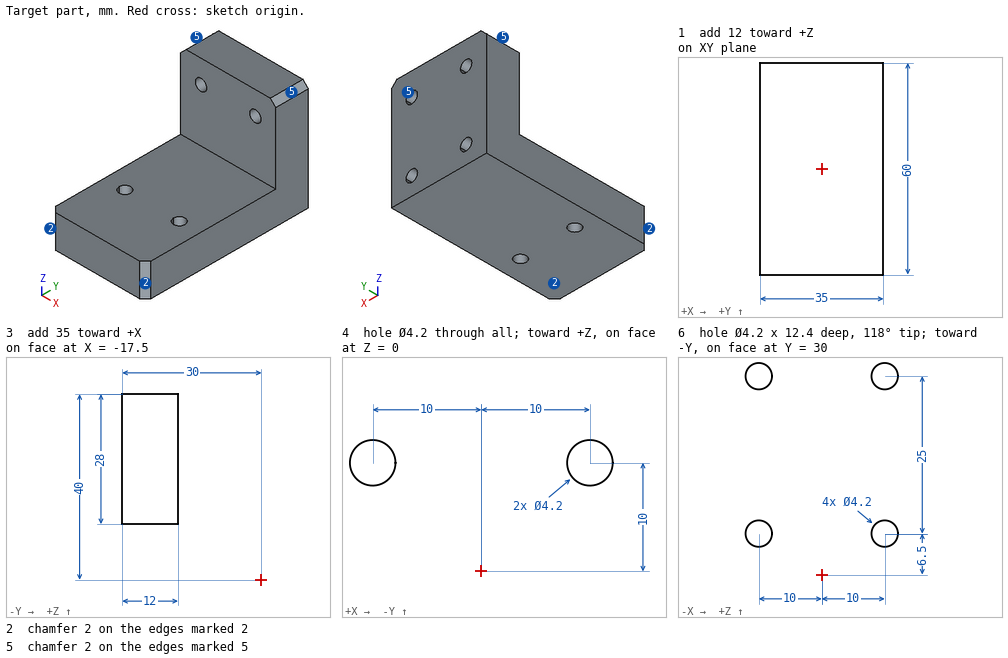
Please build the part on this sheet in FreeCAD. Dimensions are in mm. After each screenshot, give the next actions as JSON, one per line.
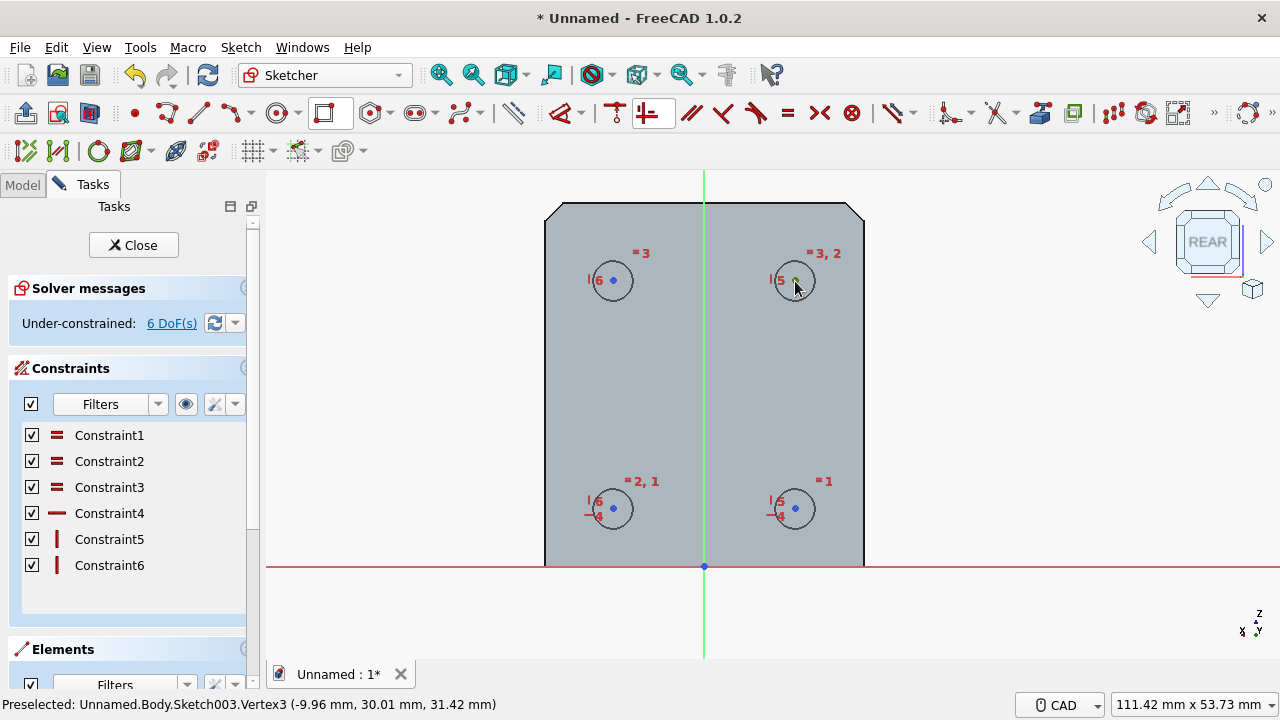
{"action": "left_click", "coordinate": [613, 281]}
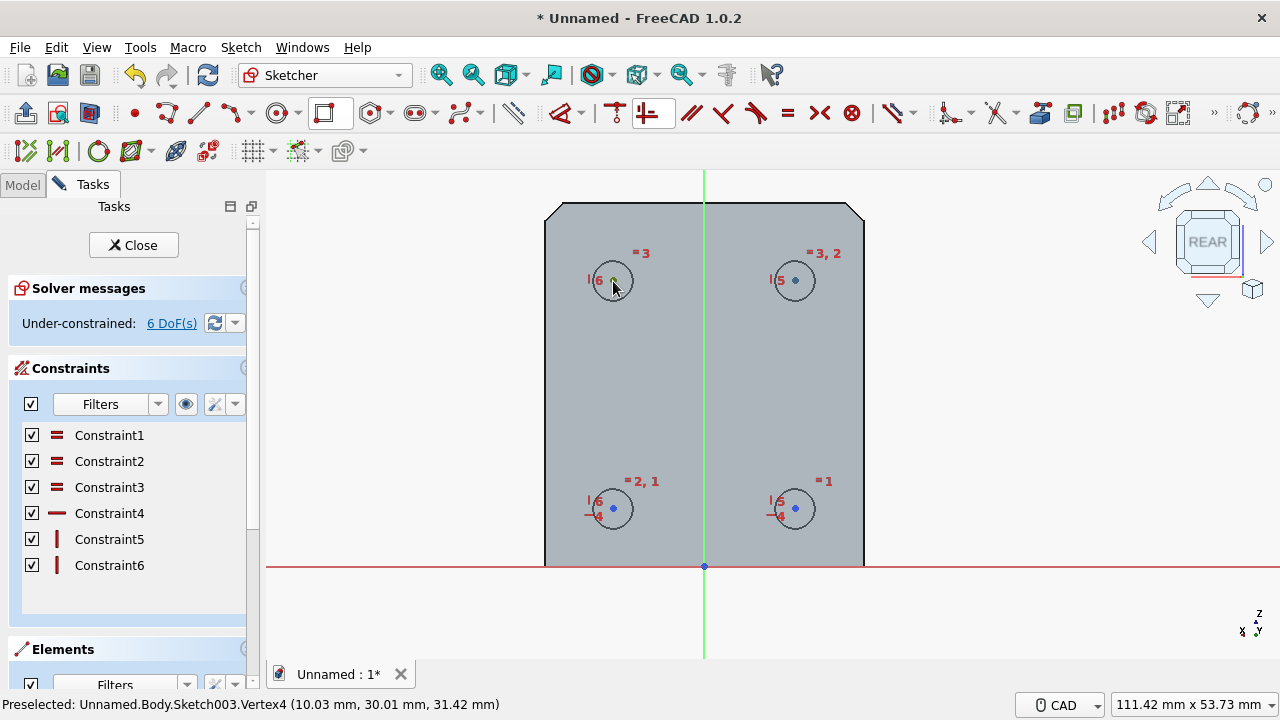
{"action": "key", "text": "h"}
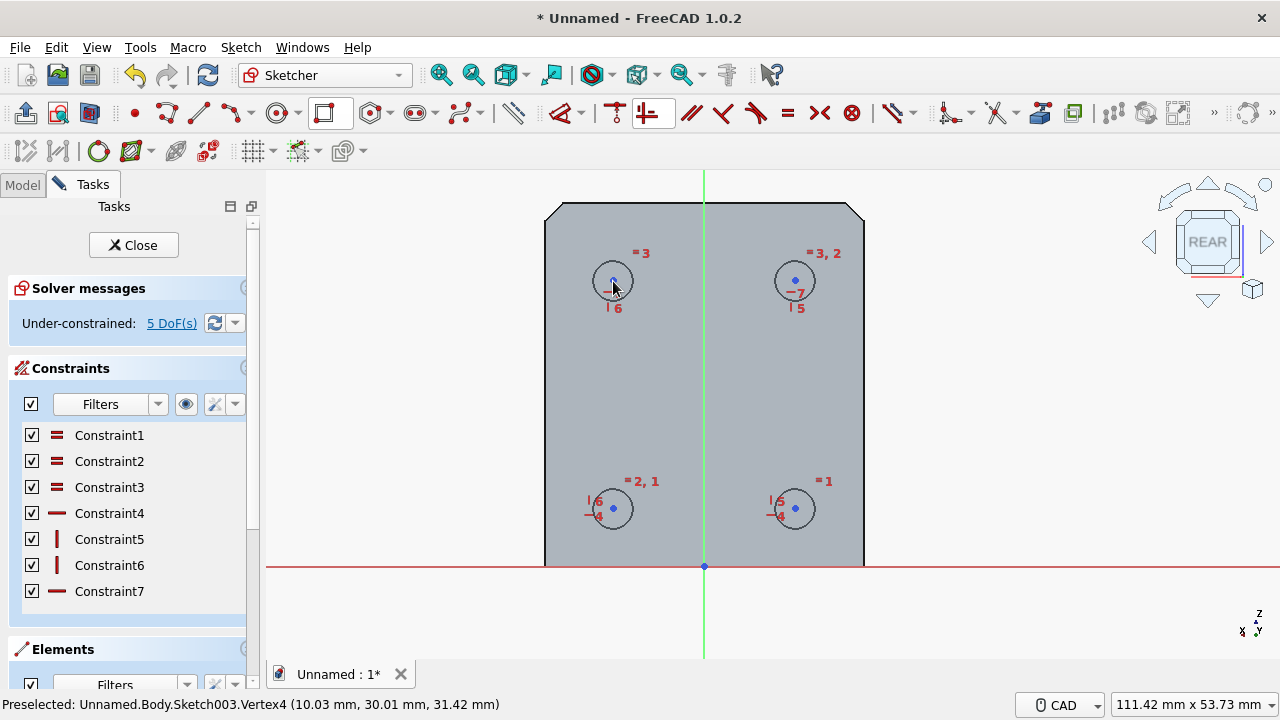
{"action": "left_click", "coordinate": [560, 114]}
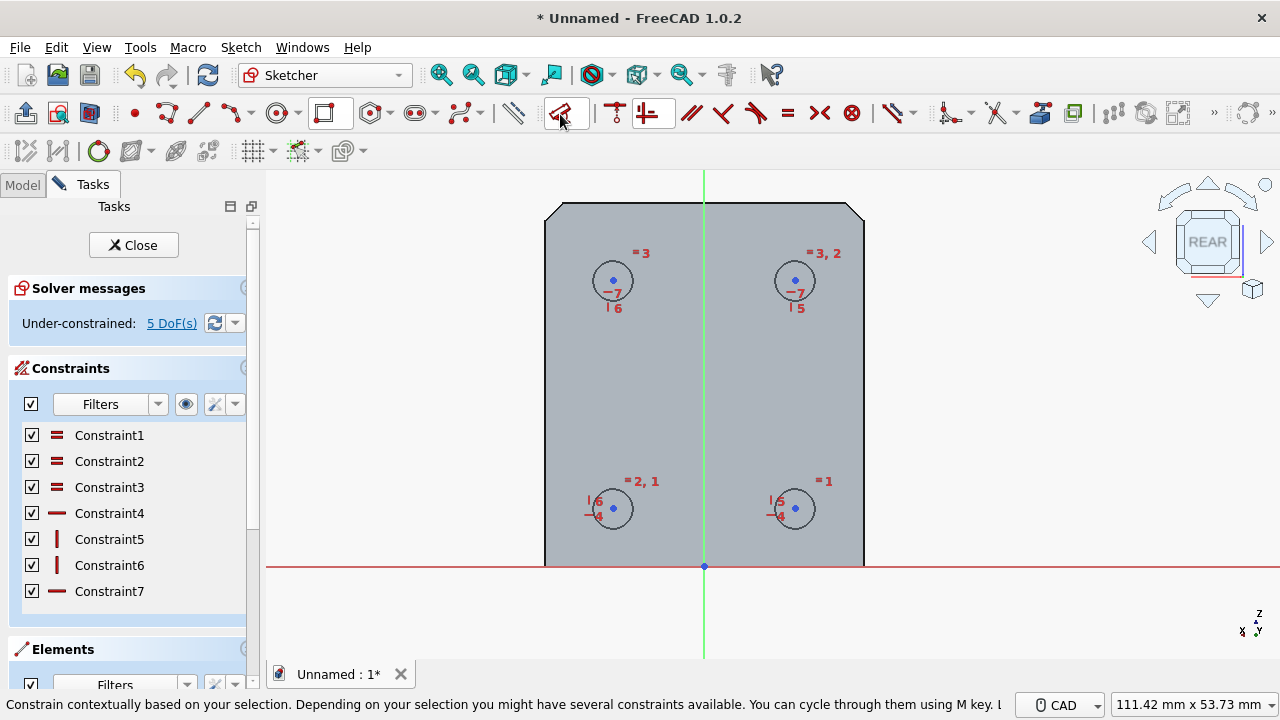
{"action": "left_click", "coordinate": [809, 495]}
{"action": "left_click", "coordinate": [832, 472]}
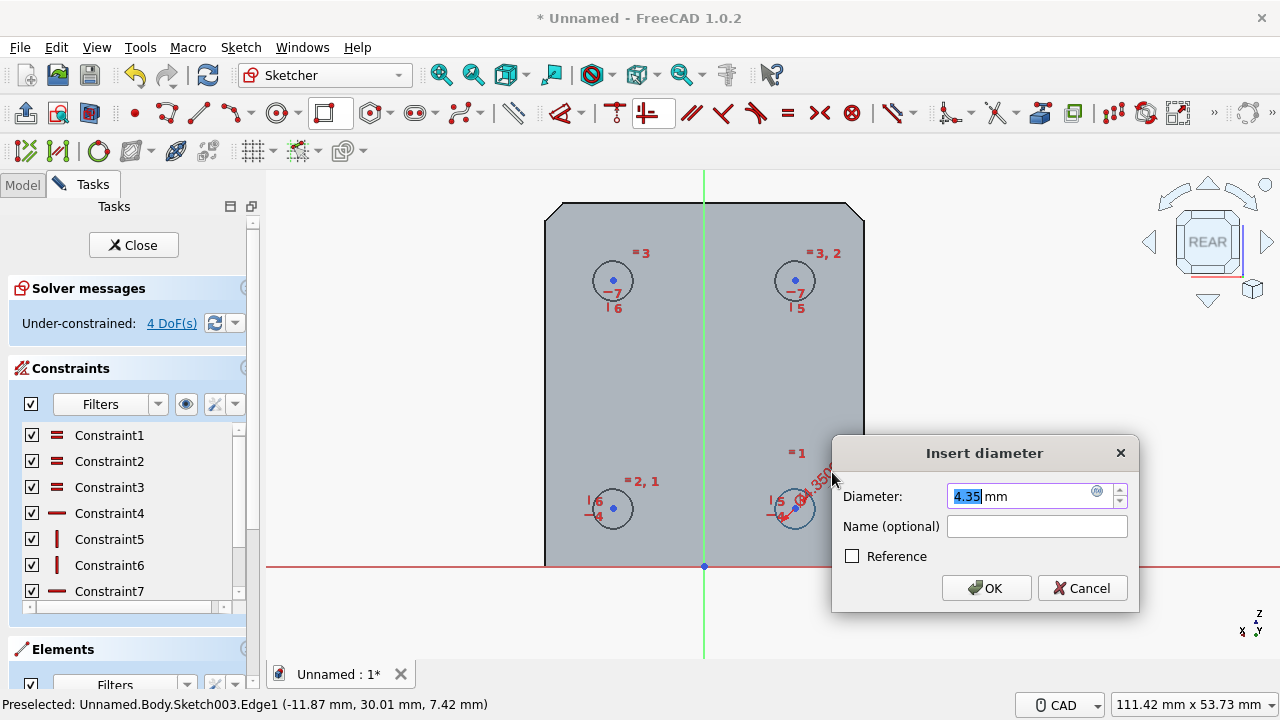
{"action": "type", "text": "4.2"}
{"action": "key", "text": "Return"}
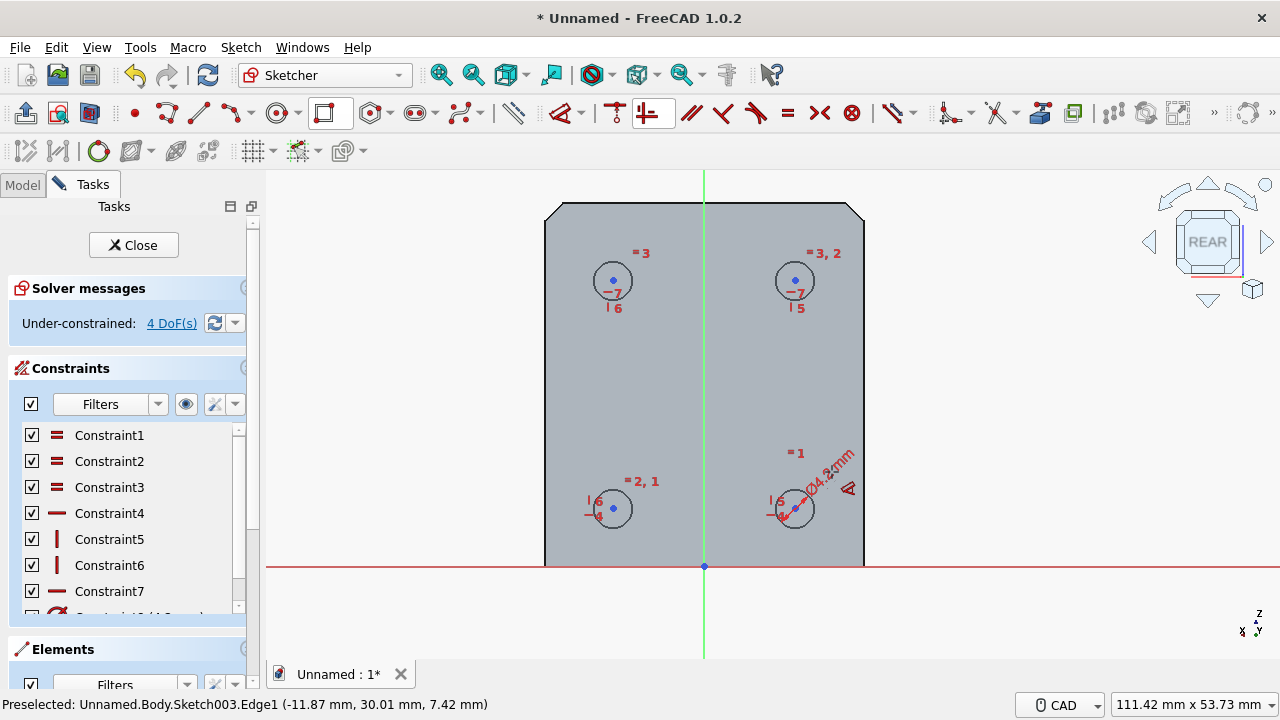
{"action": "left_click", "coordinate": [795, 509]}
{"action": "left_click", "coordinate": [750, 601]}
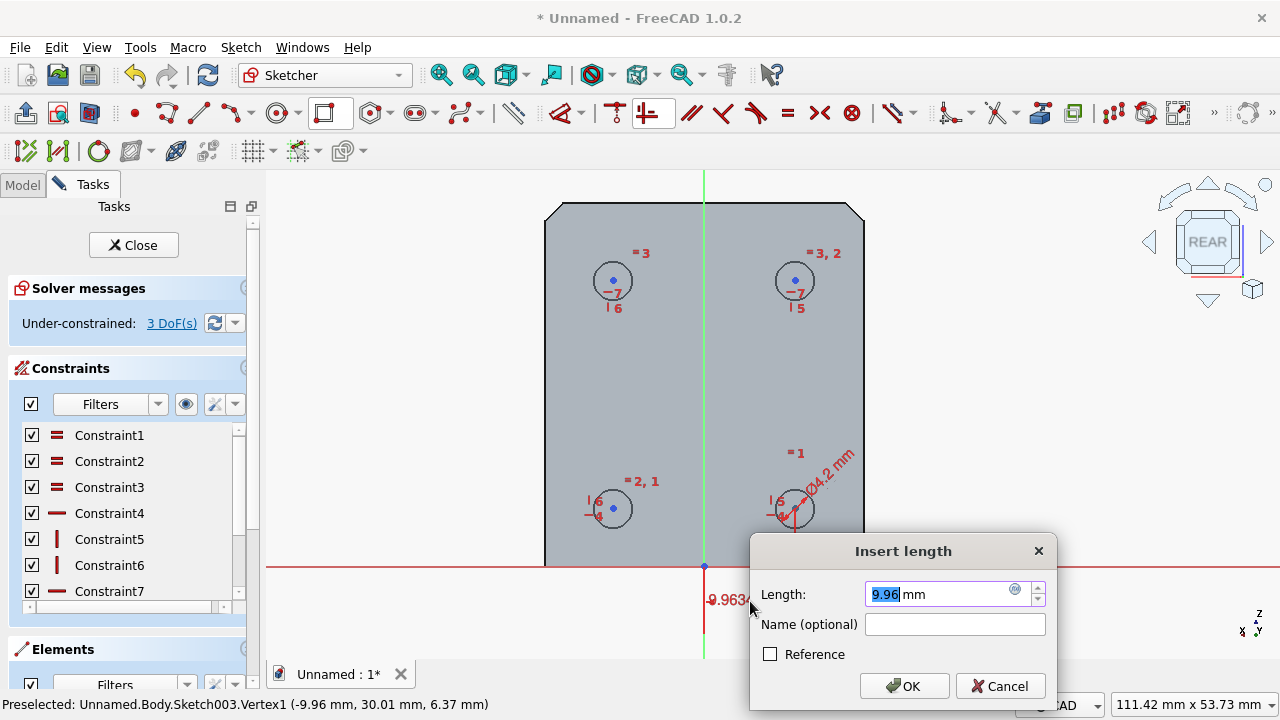
{"action": "type", "text": "10"}
{"action": "key", "text": "Return"}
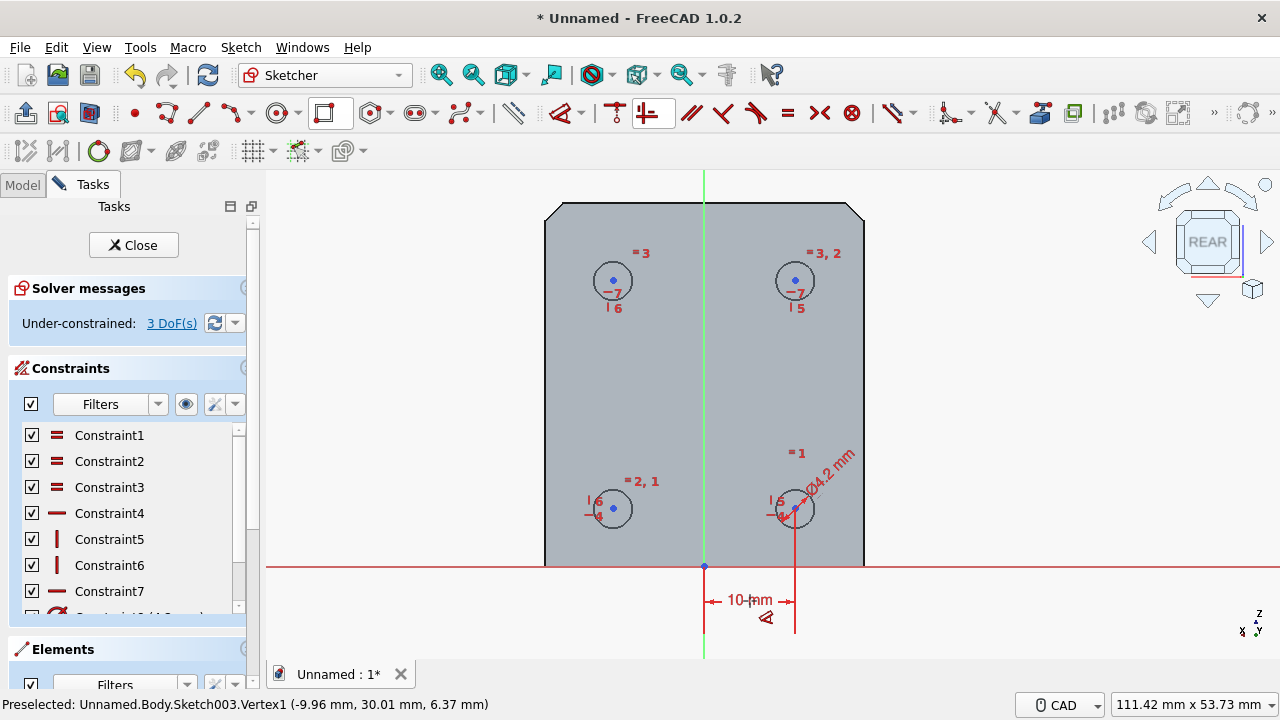
{"action": "left_click", "coordinate": [613, 509]}
{"action": "left_click", "coordinate": [659, 601]}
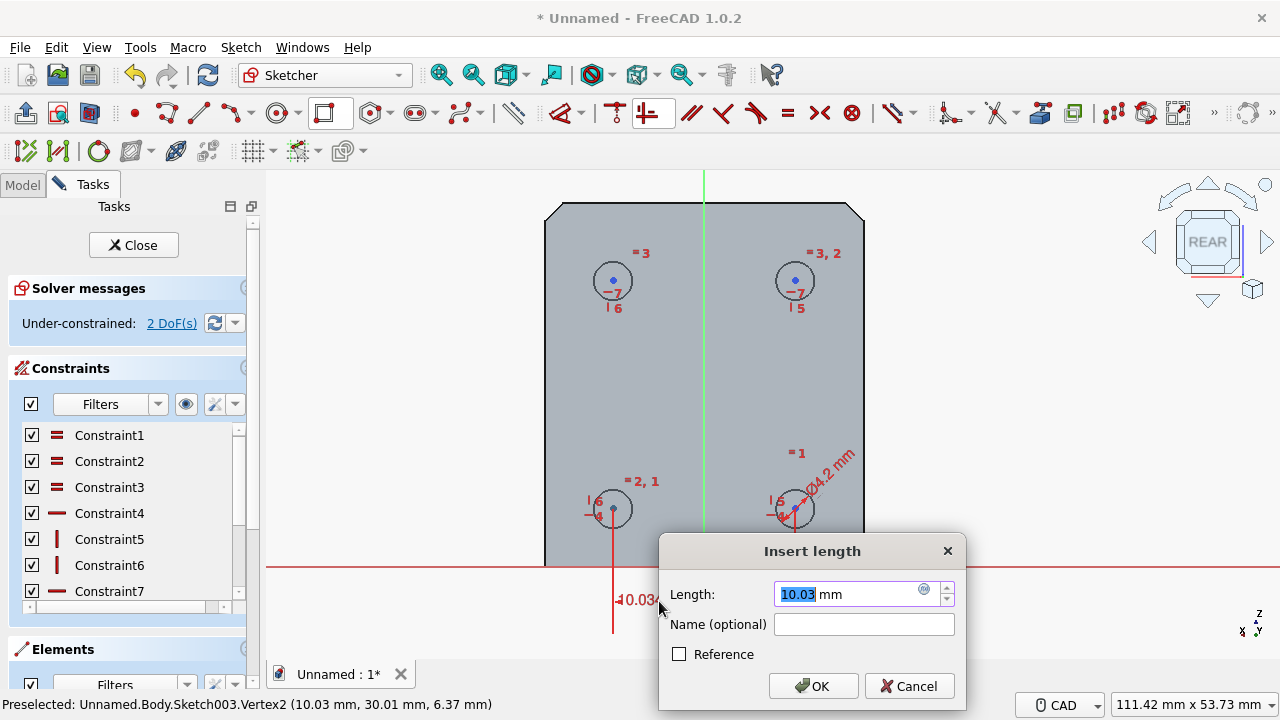
{"action": "type", "text": "10"}
{"action": "key", "text": "Return"}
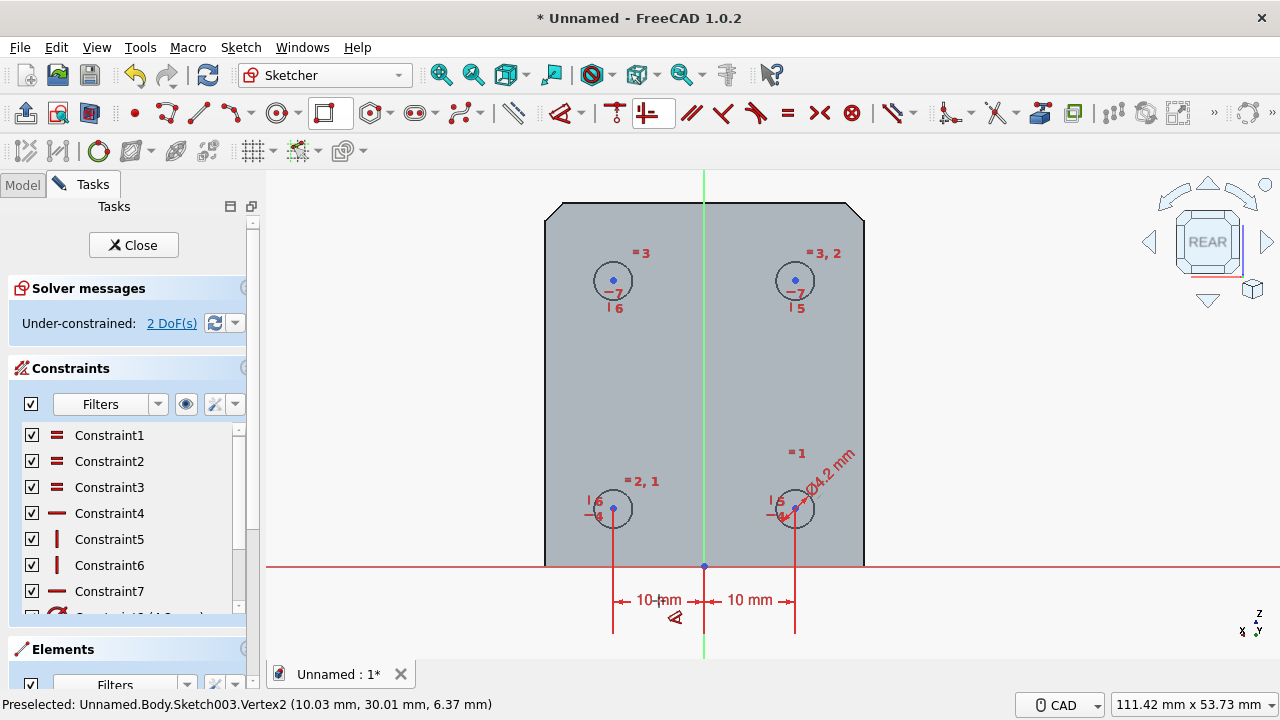
{"action": "left_click", "coordinate": [795, 509]}
{"action": "left_click", "coordinate": [829, 538]}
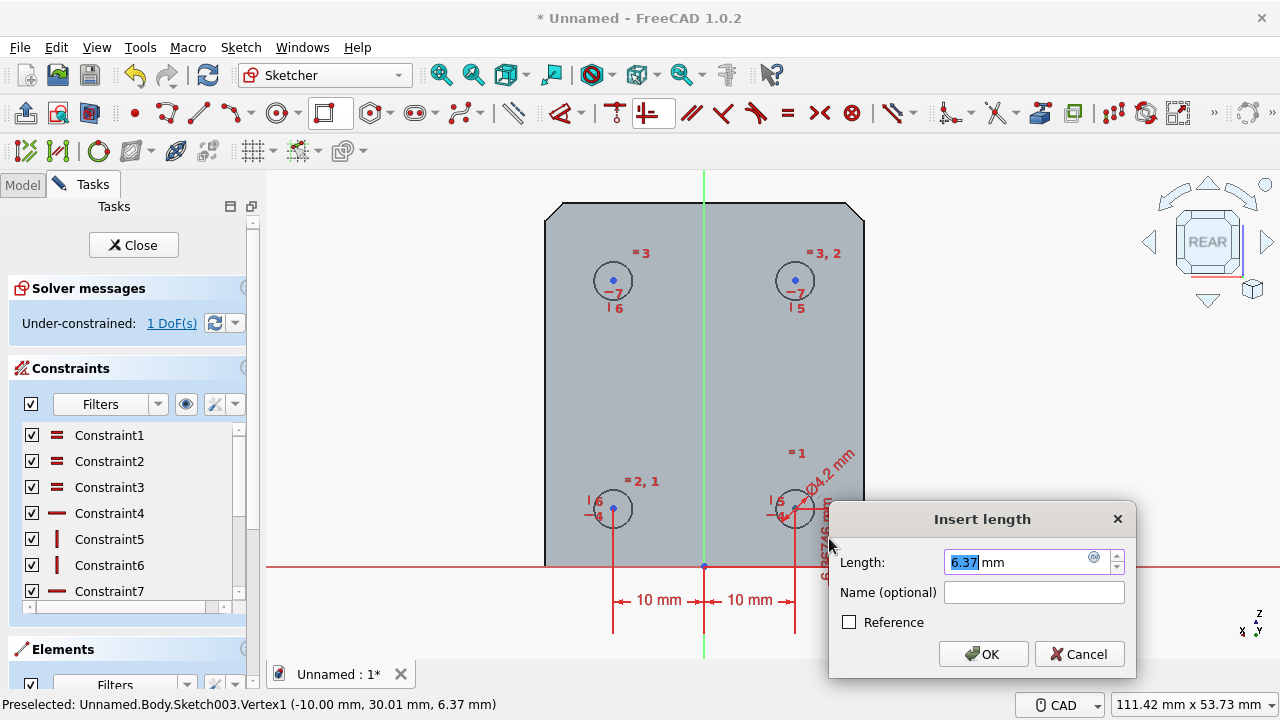
{"action": "type", "text": "6.5"}
{"action": "key", "text": "Return"}